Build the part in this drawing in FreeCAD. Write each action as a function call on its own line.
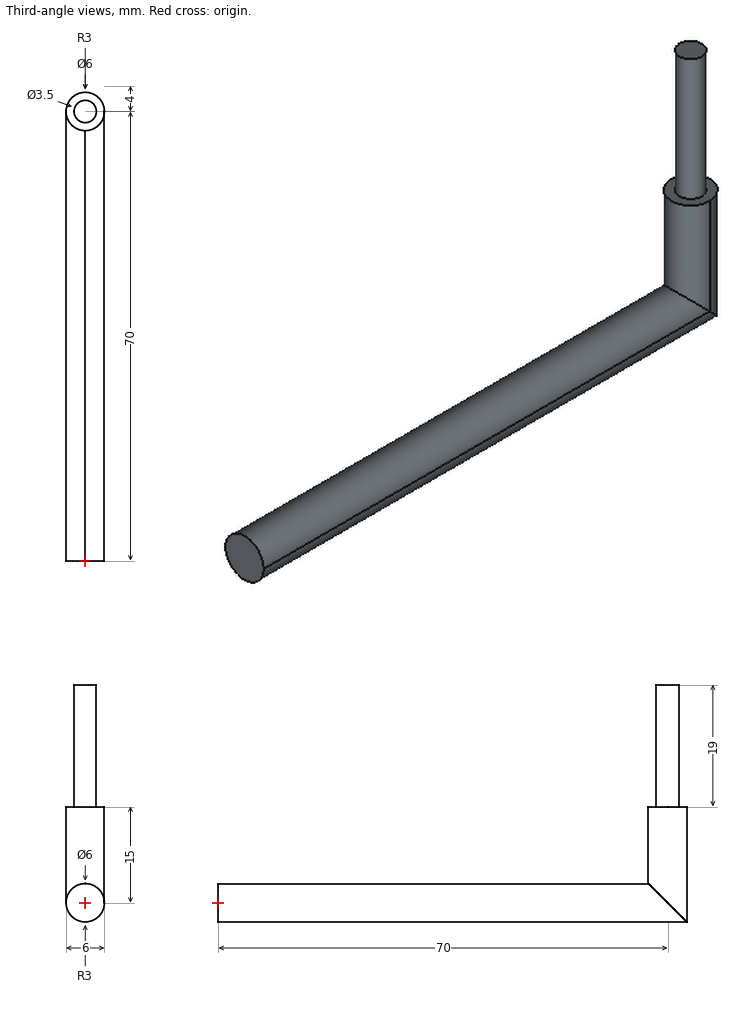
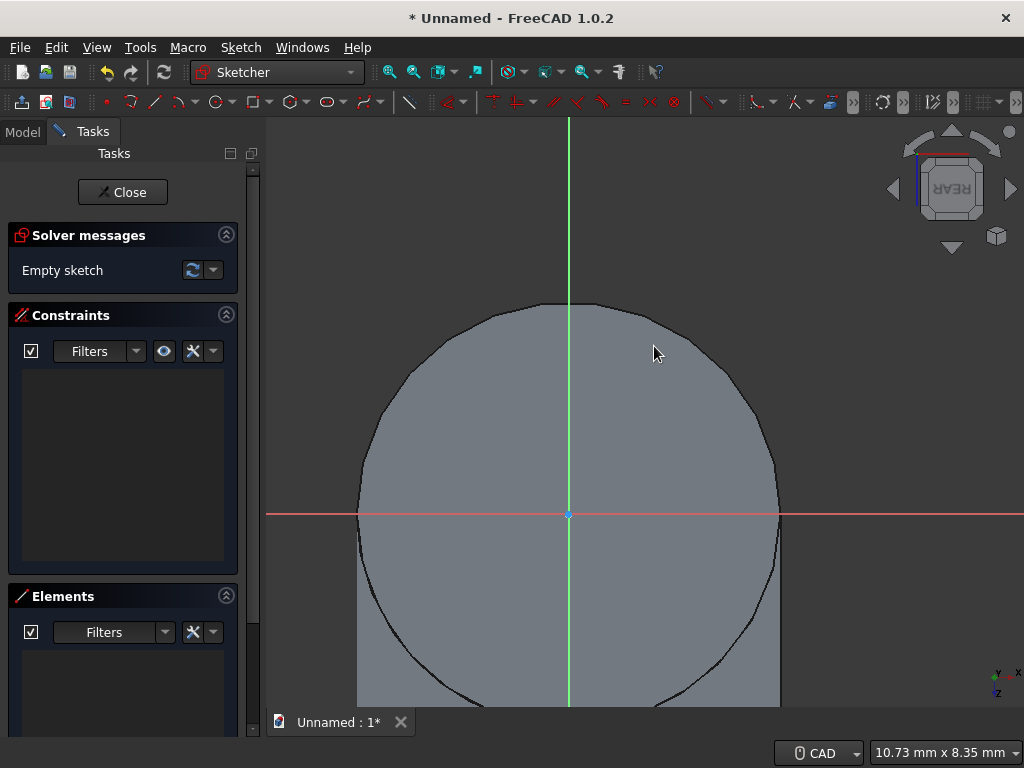
click(156, 102)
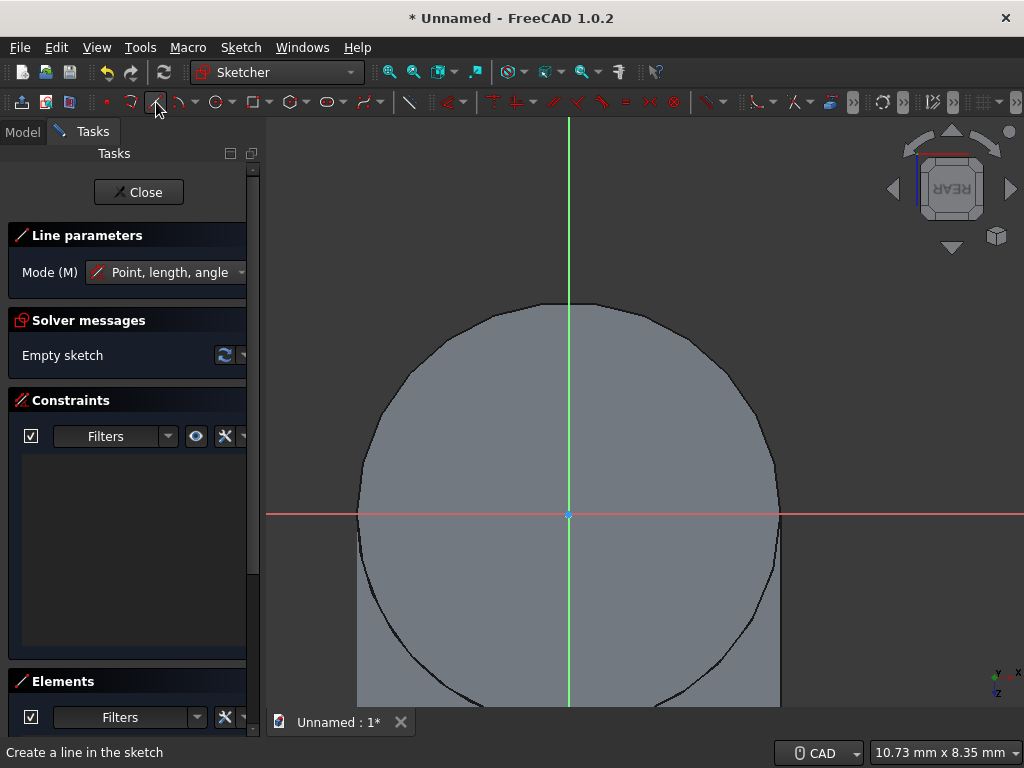
click(357, 514)
click(781, 505)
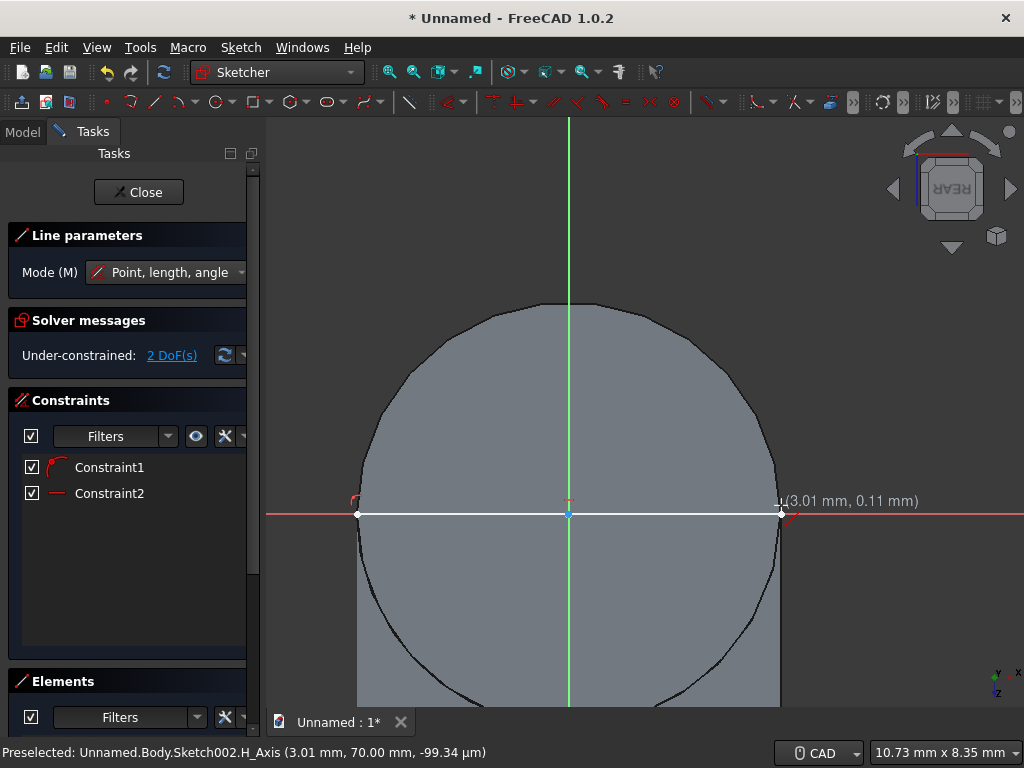
key(g)
key(3)
key(a)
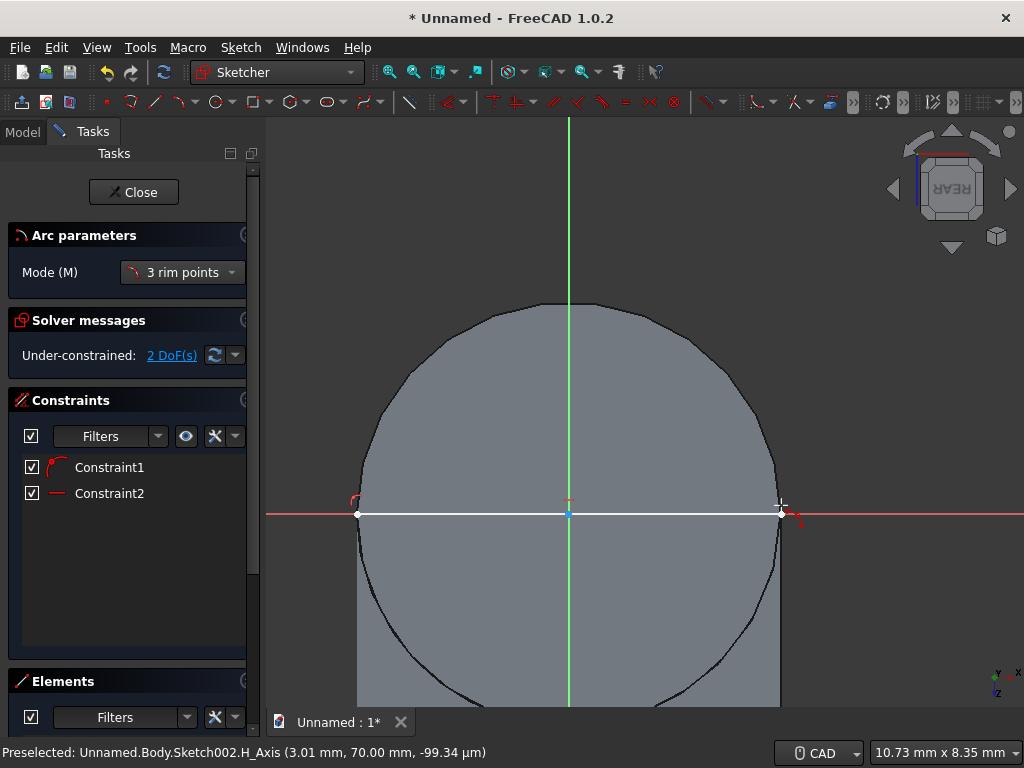
click(781, 505)
click(357, 514)
click(634, 313)
key(Escape)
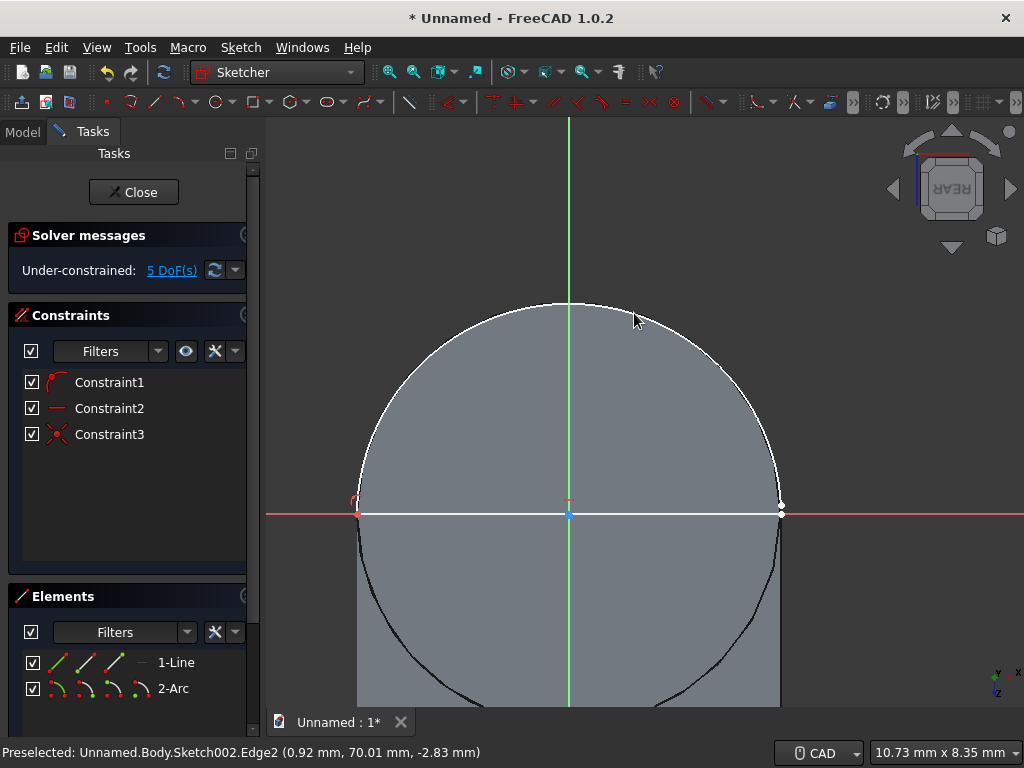
drag(559, 504, 579, 526)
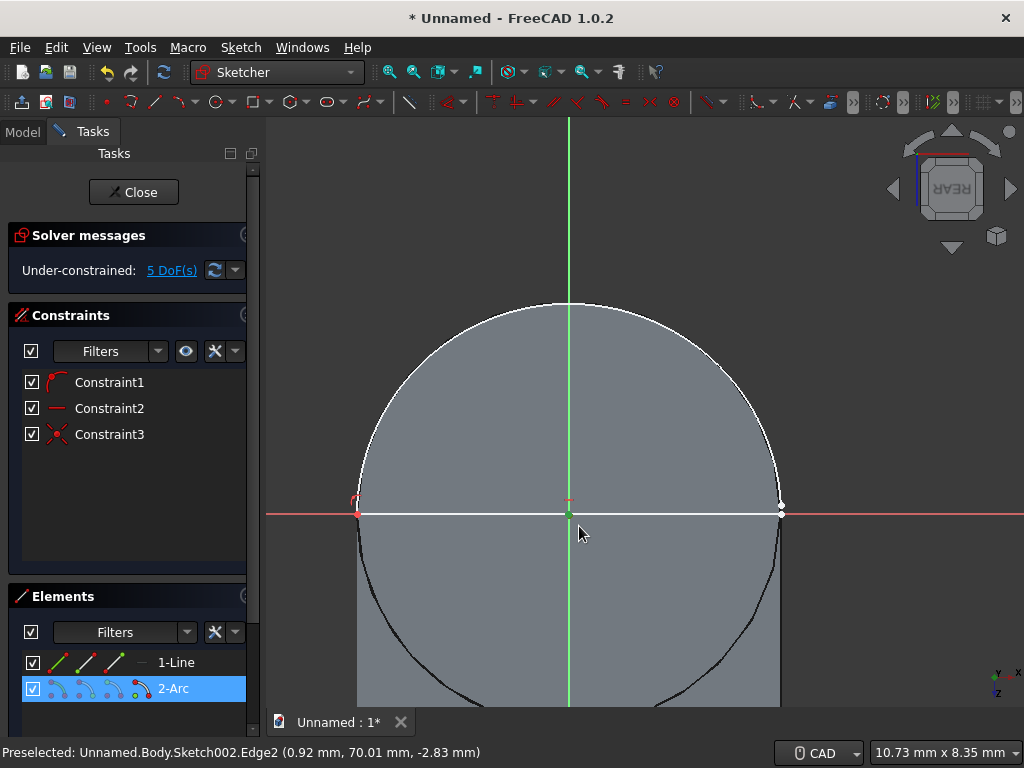
click(494, 102)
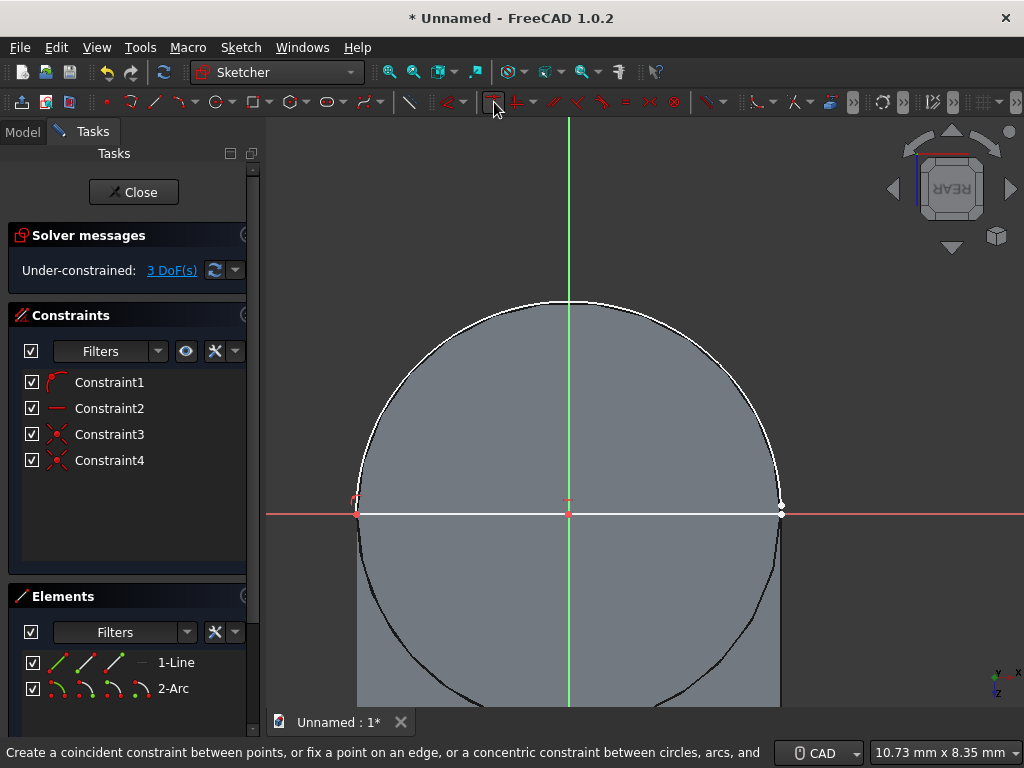
click(448, 102)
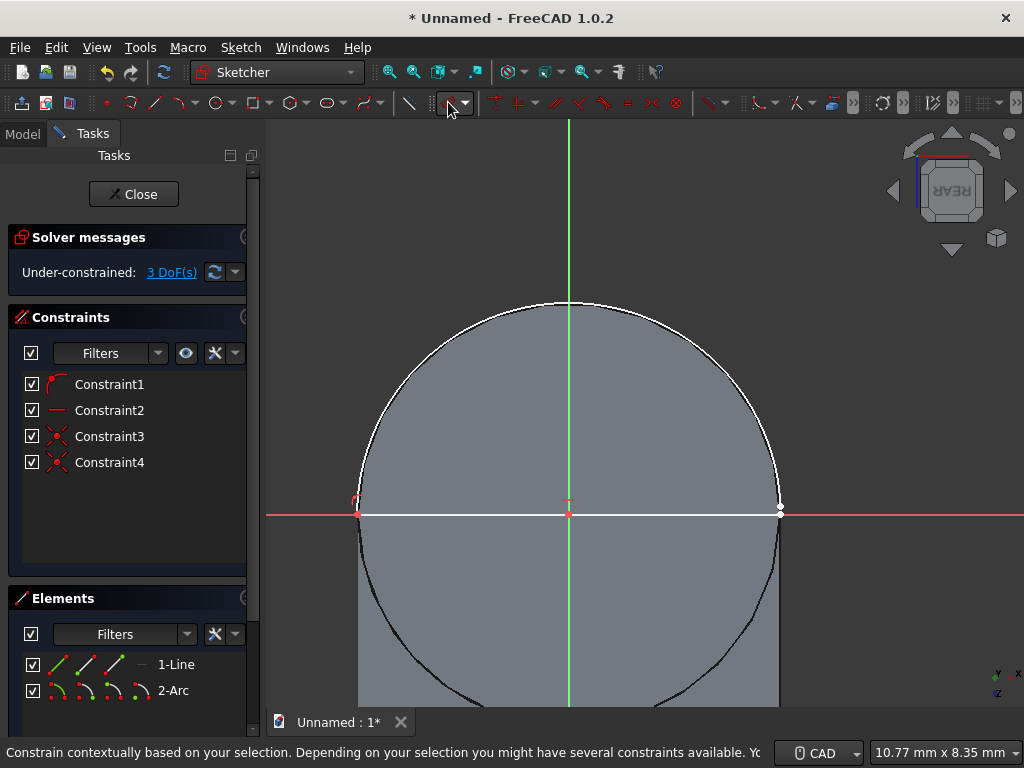
click(689, 340)
click(707, 314)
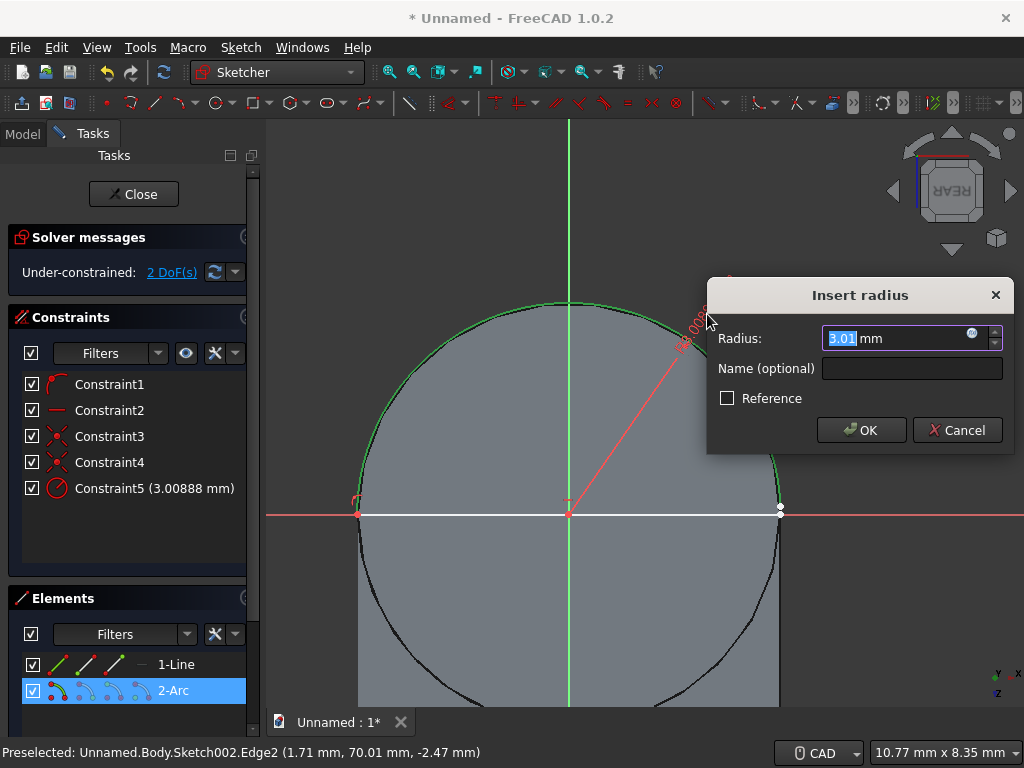
text(3)
key(Return)
key(Escape)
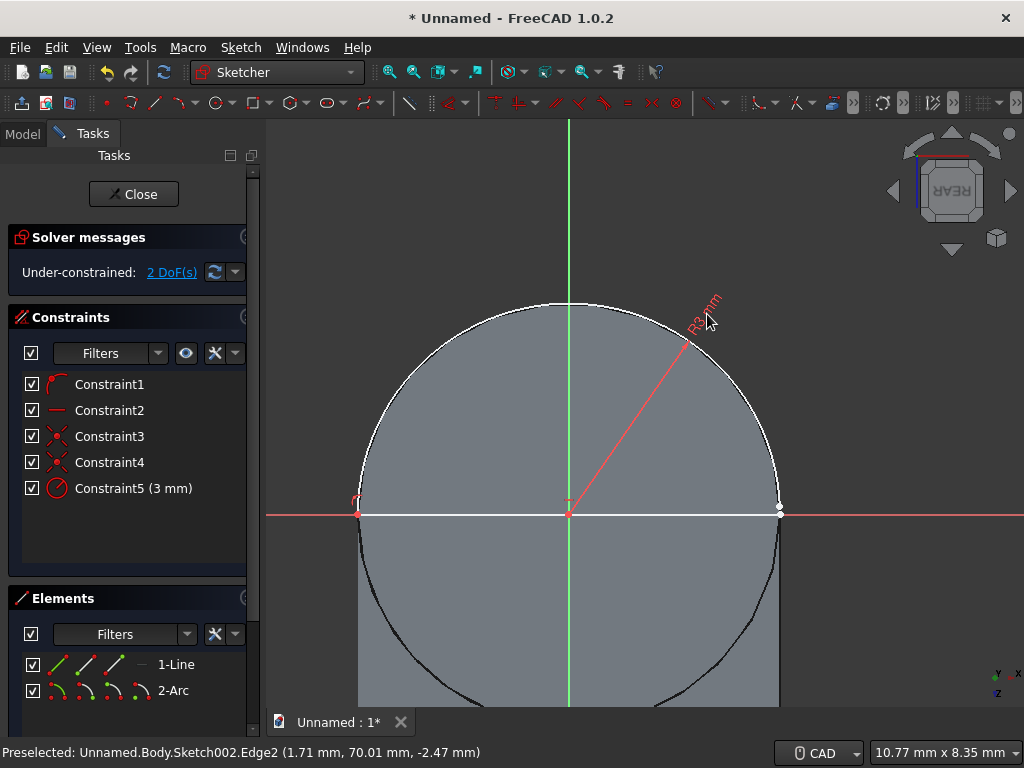
click(780, 507)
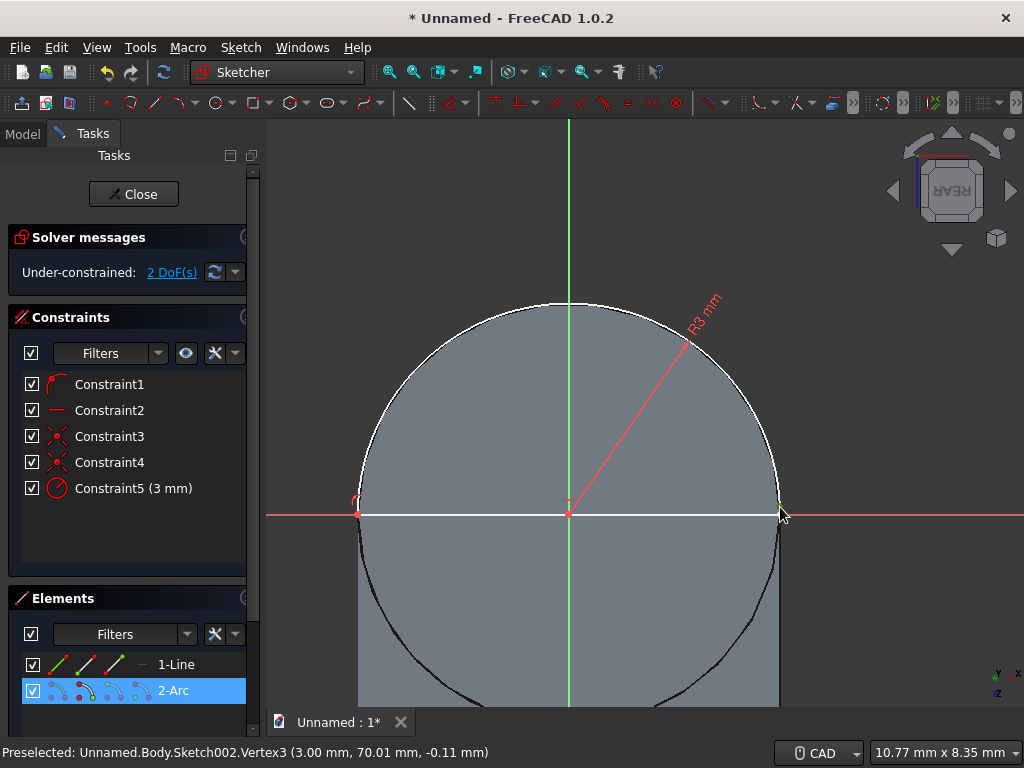
click(819, 515)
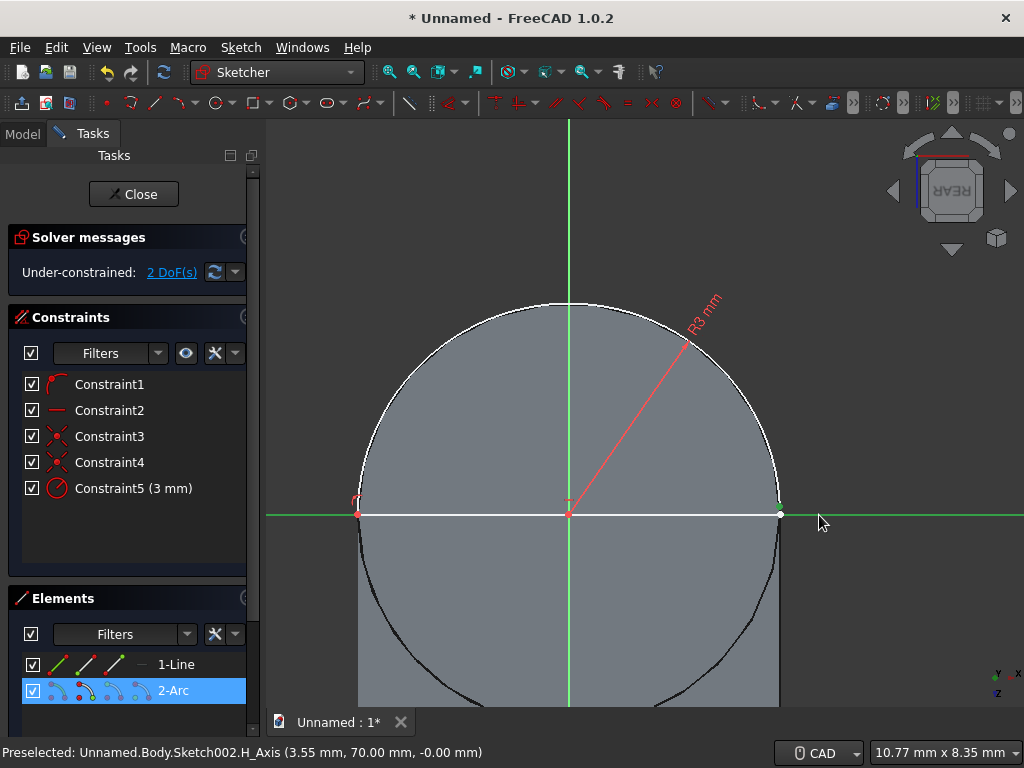
key(c)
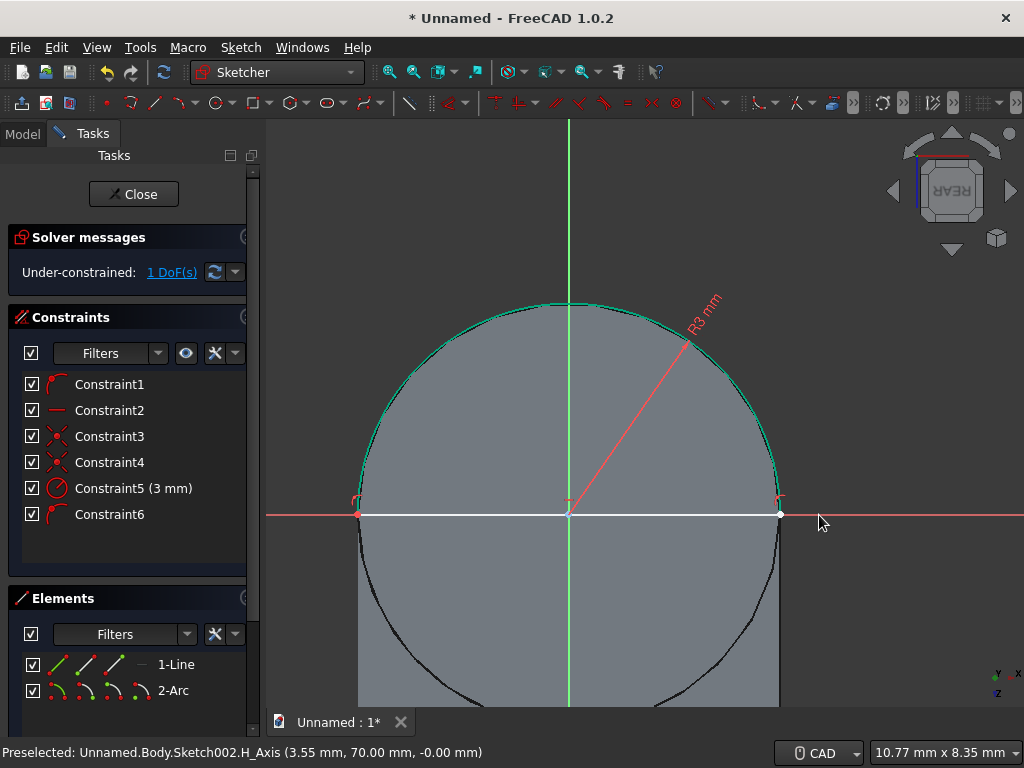
key(d)